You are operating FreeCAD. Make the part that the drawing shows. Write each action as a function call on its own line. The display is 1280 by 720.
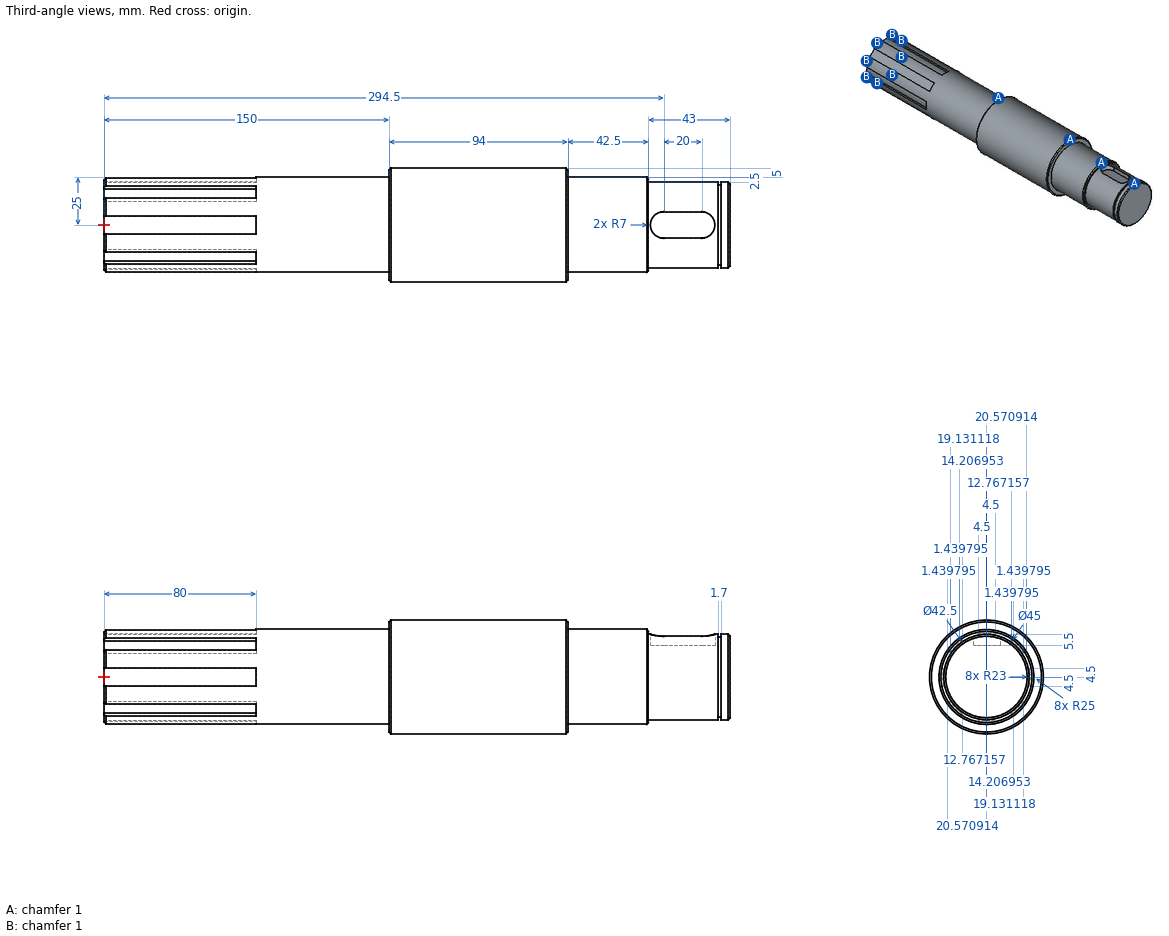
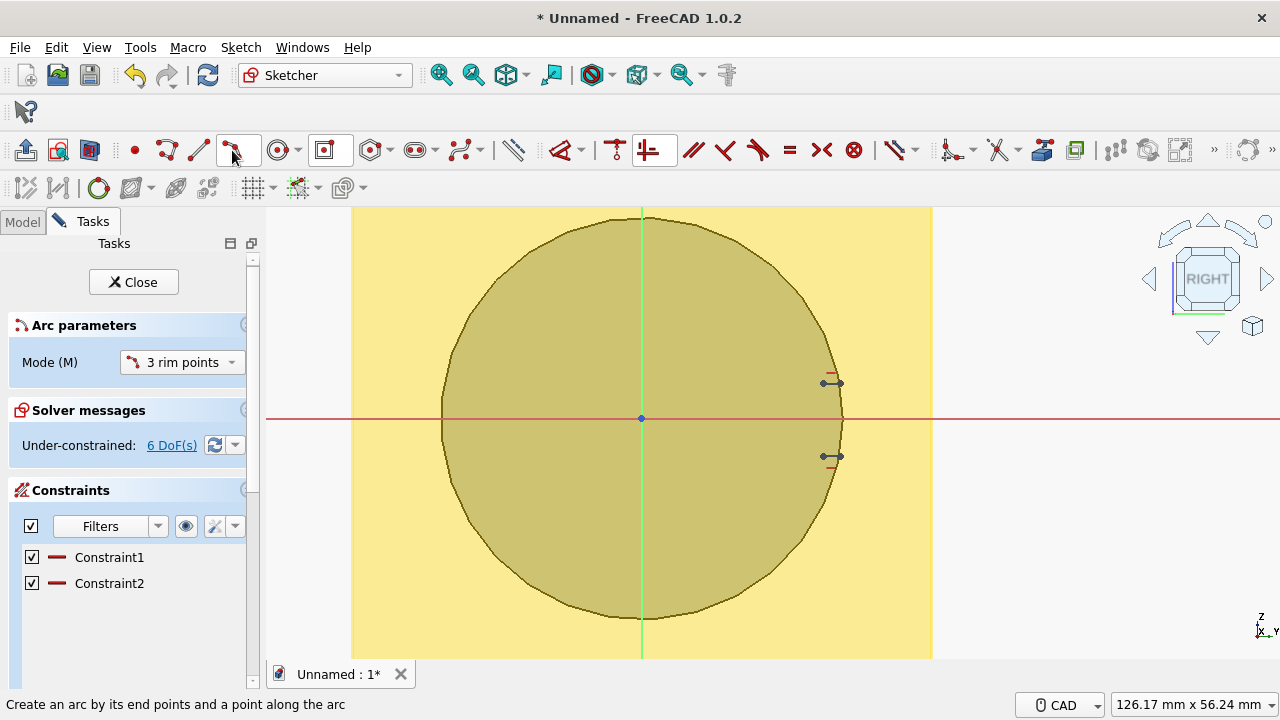
scroll(823, 455, up, 4)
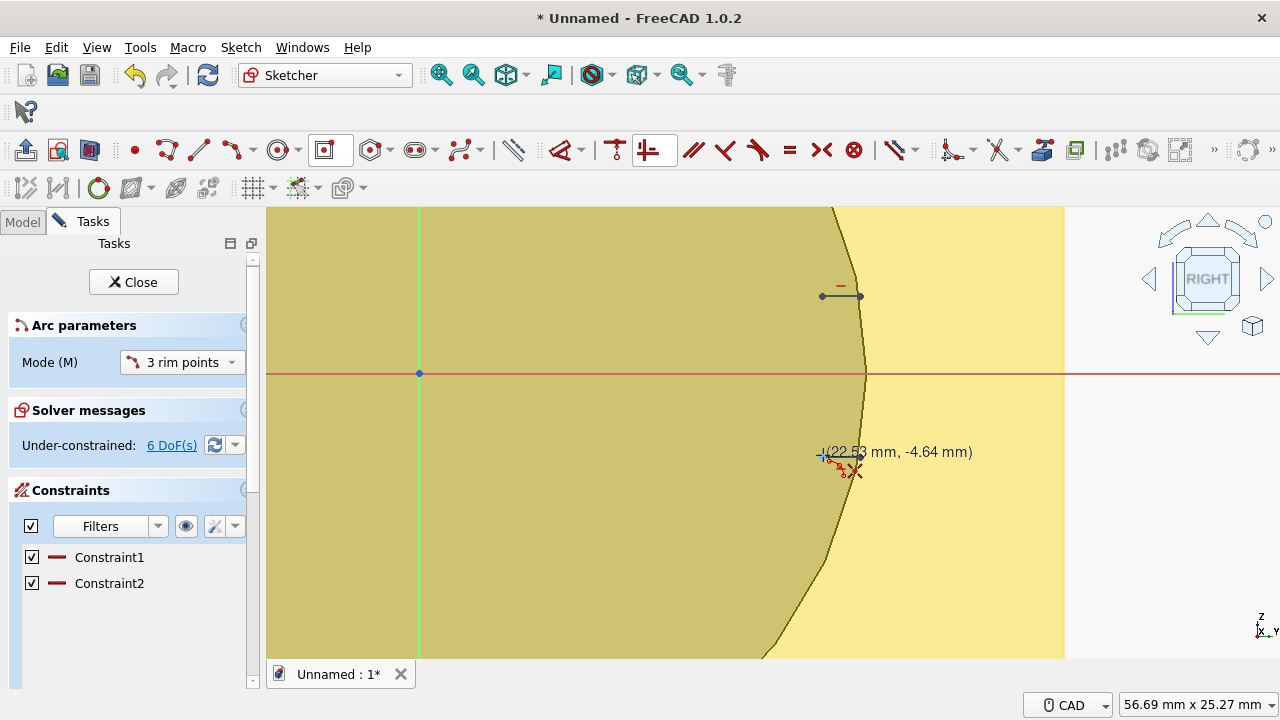
click(822, 457)
click(822, 296)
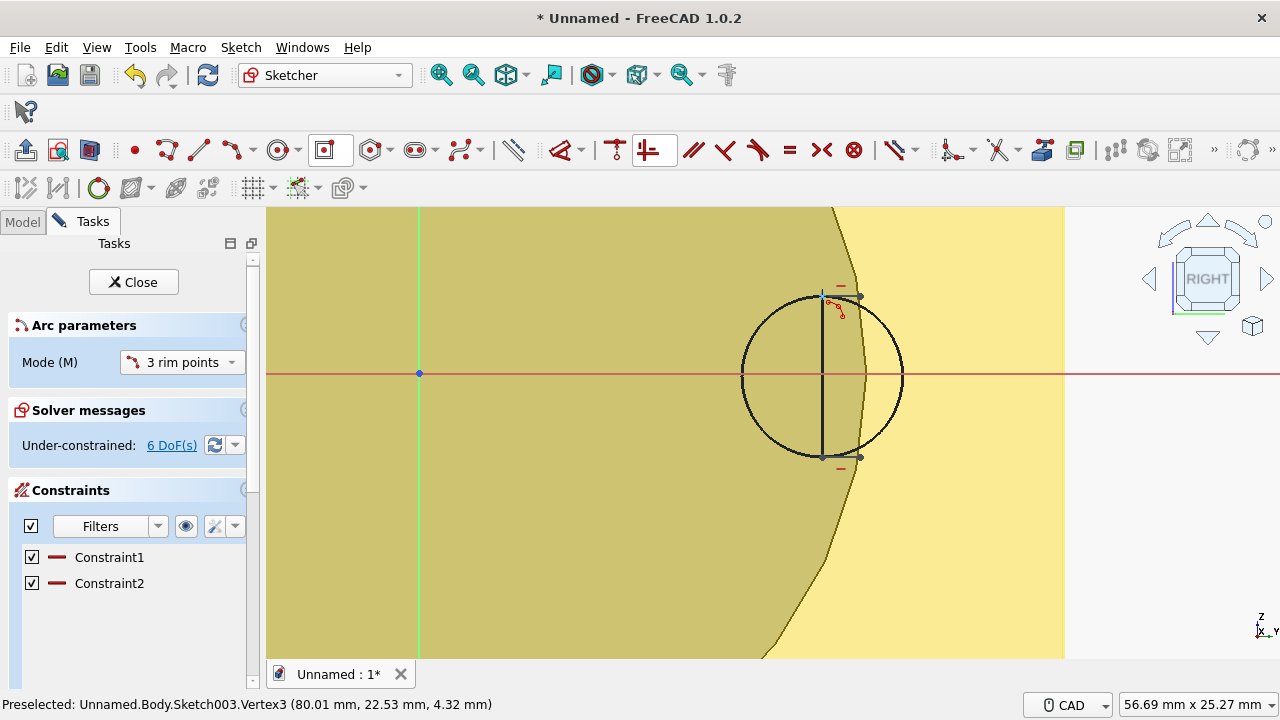
scroll(830, 390, up, 4)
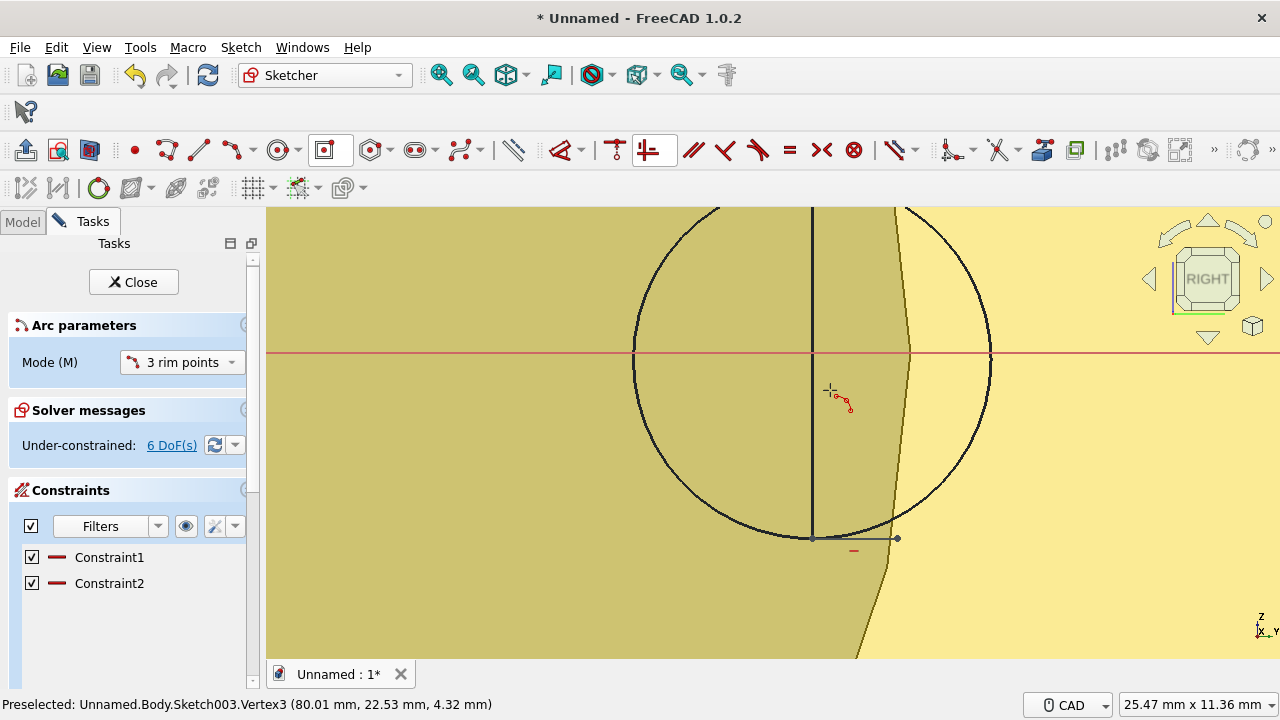
click(830, 389)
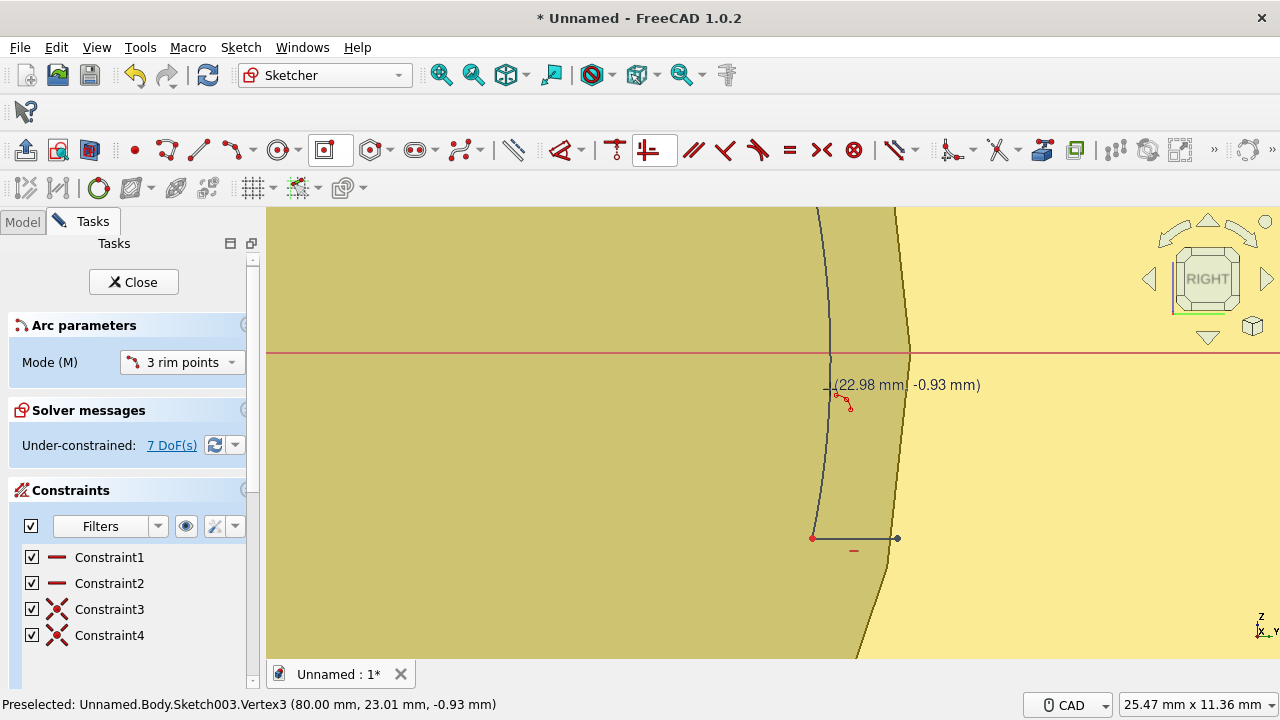
scroll(828, 446, down, 10)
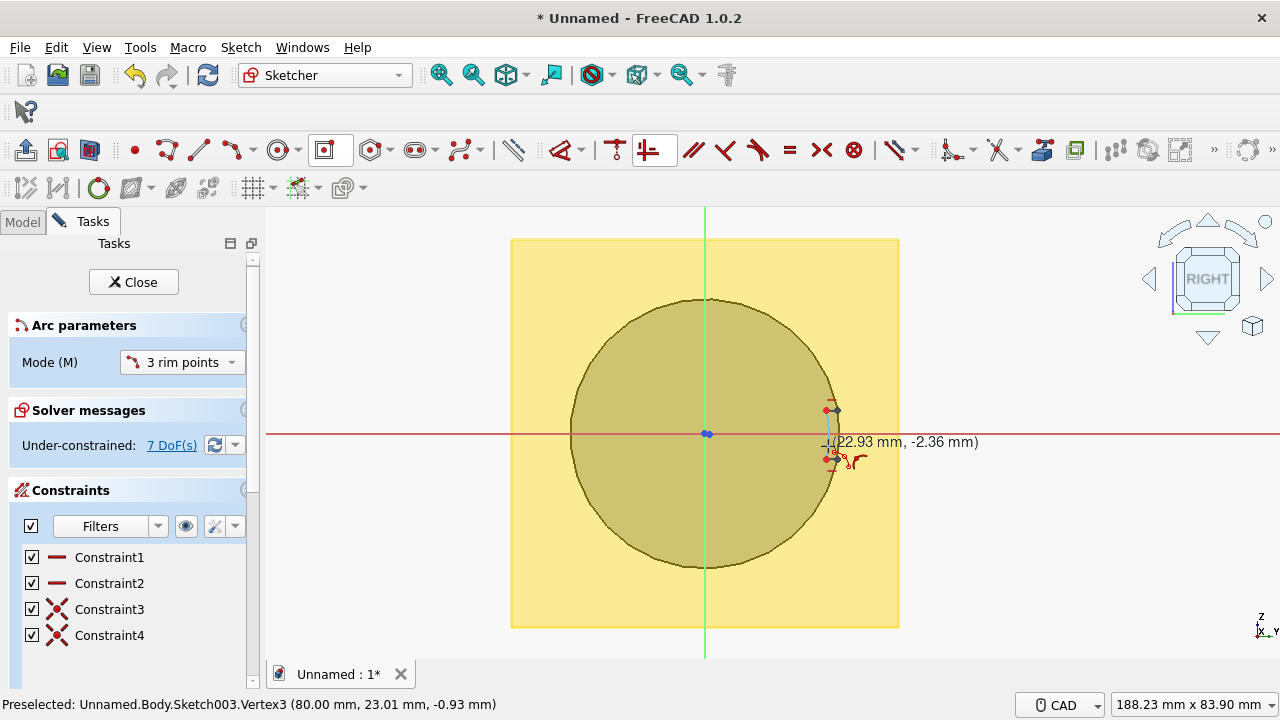
scroll(837, 410, up, 6)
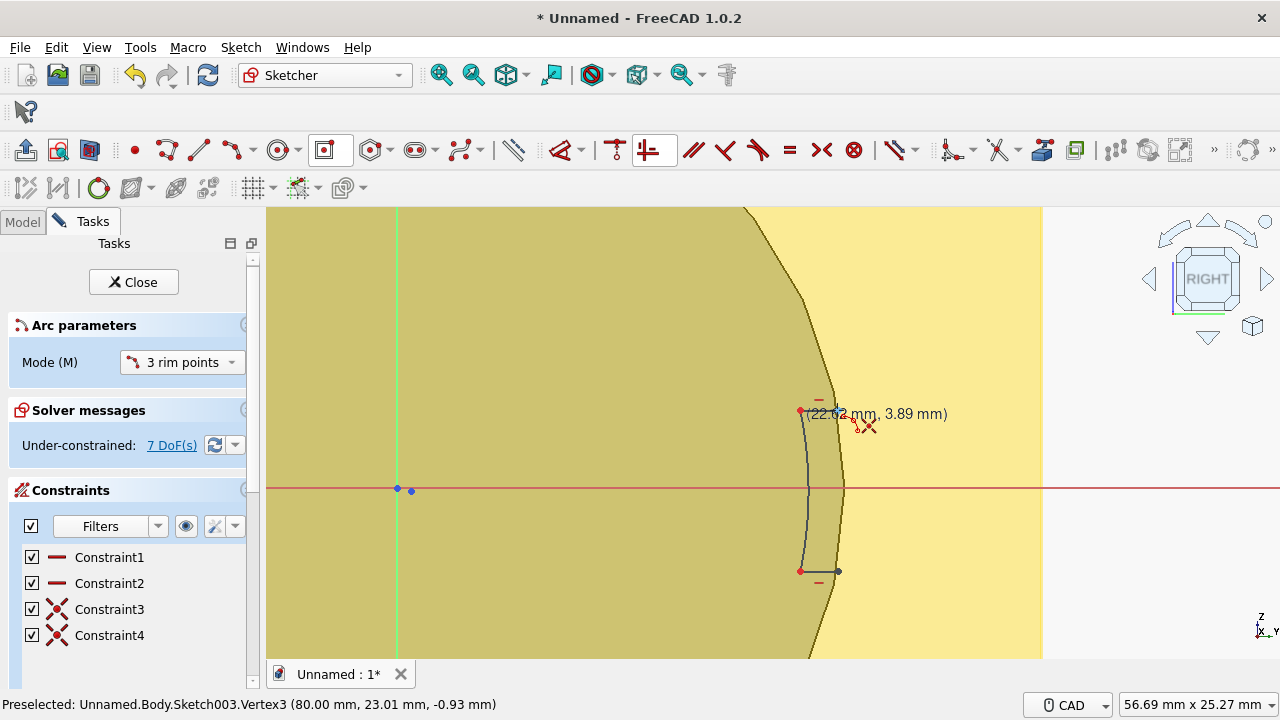
click(838, 411)
click(838, 572)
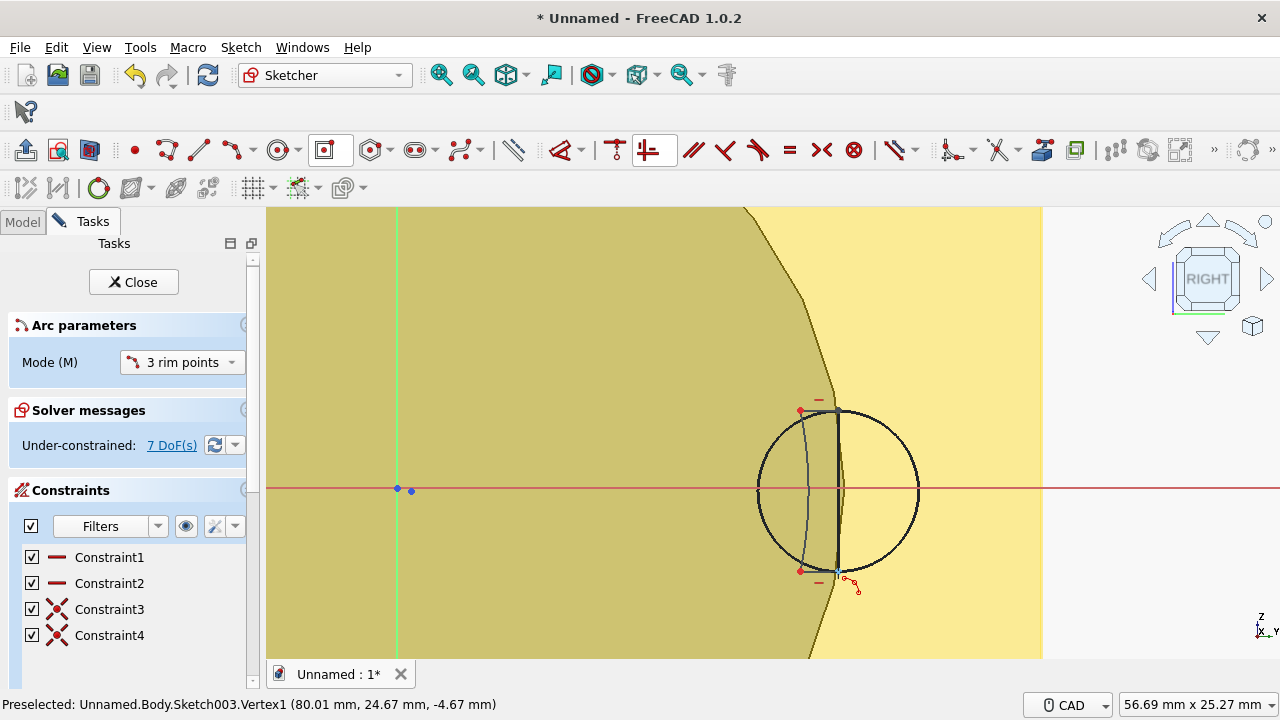
scroll(844, 504, up, 5)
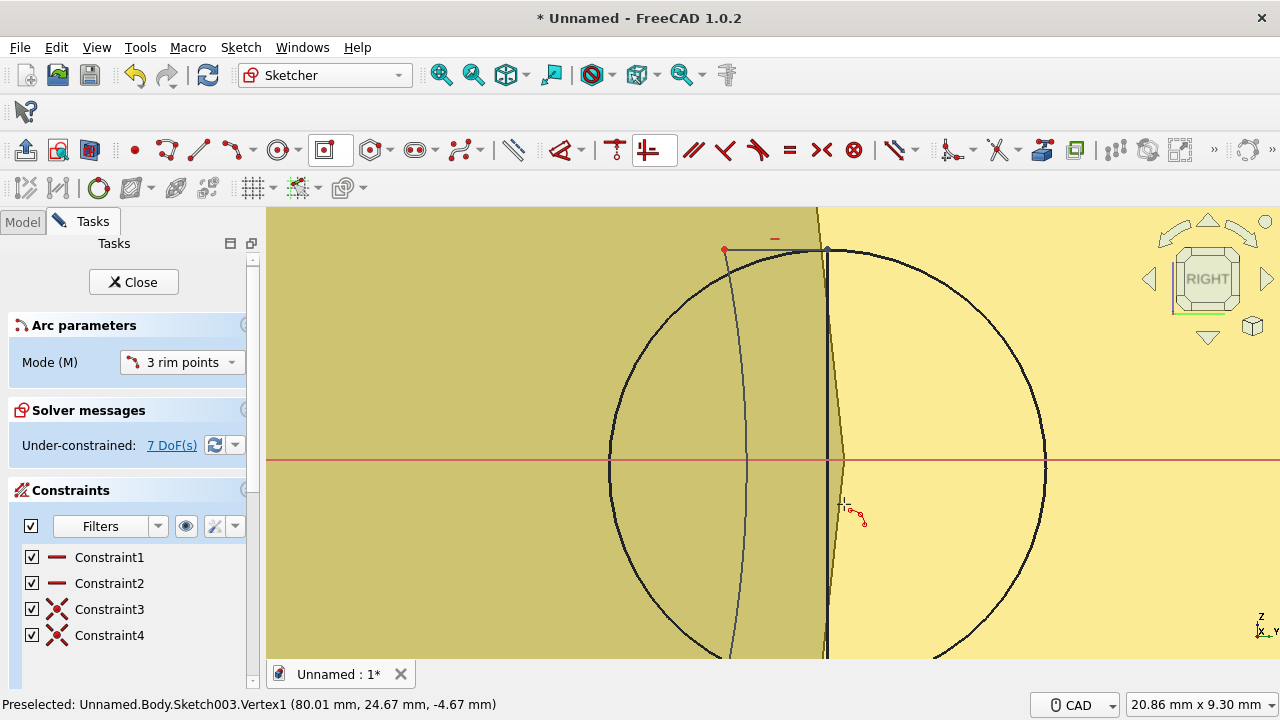
click(843, 504)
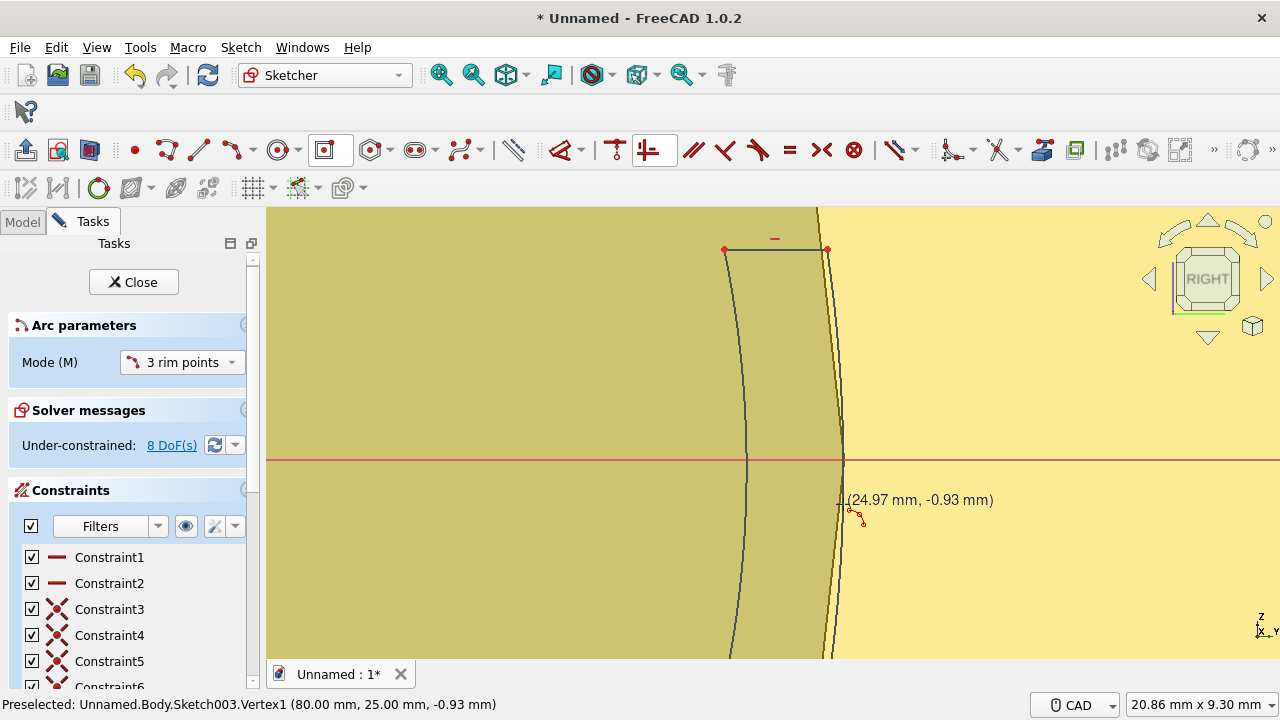
click(200, 150)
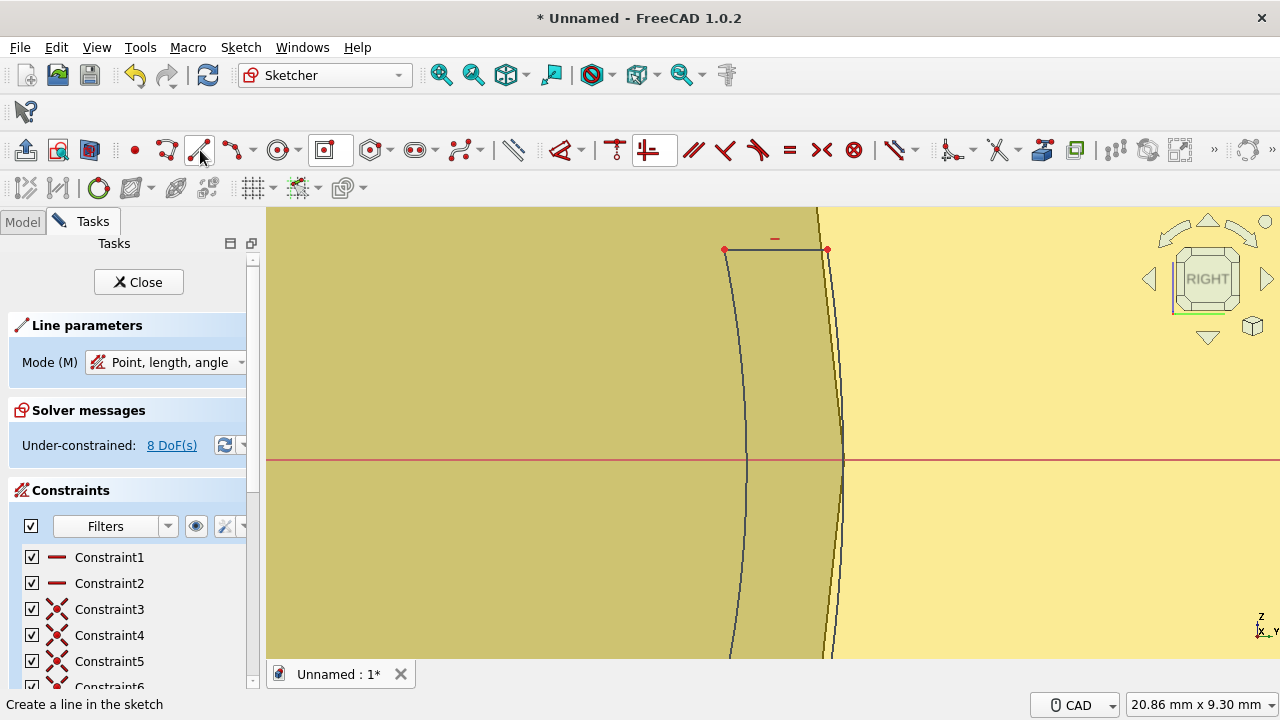
scroll(839, 430, down, 11)